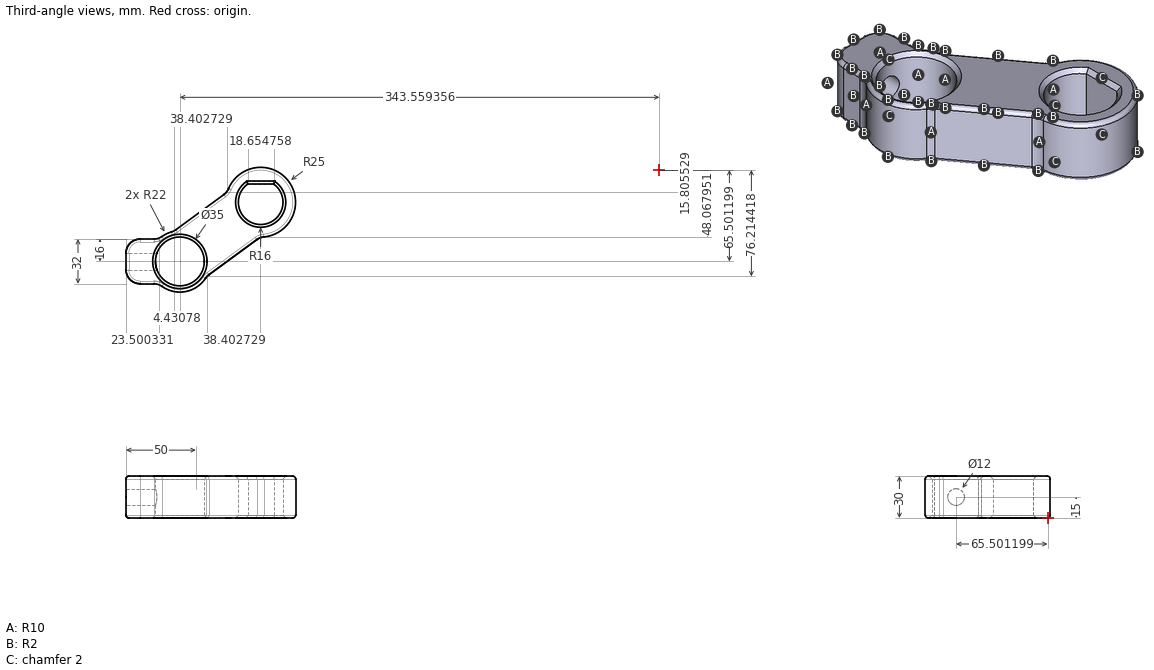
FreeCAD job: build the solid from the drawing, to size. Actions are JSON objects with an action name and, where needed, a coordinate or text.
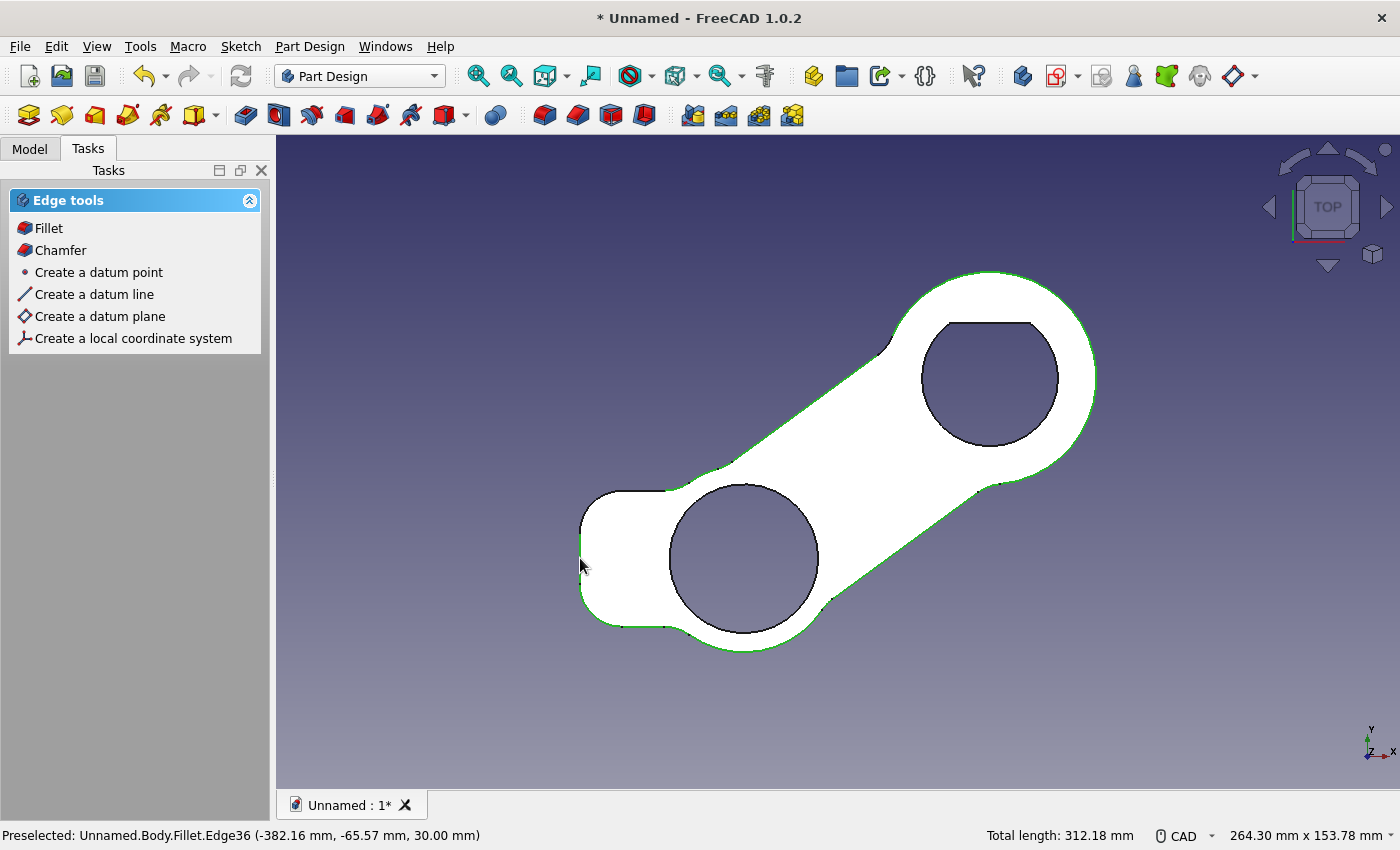
{"action": "left_click", "coordinate": [643, 490], "text": "ctrl"}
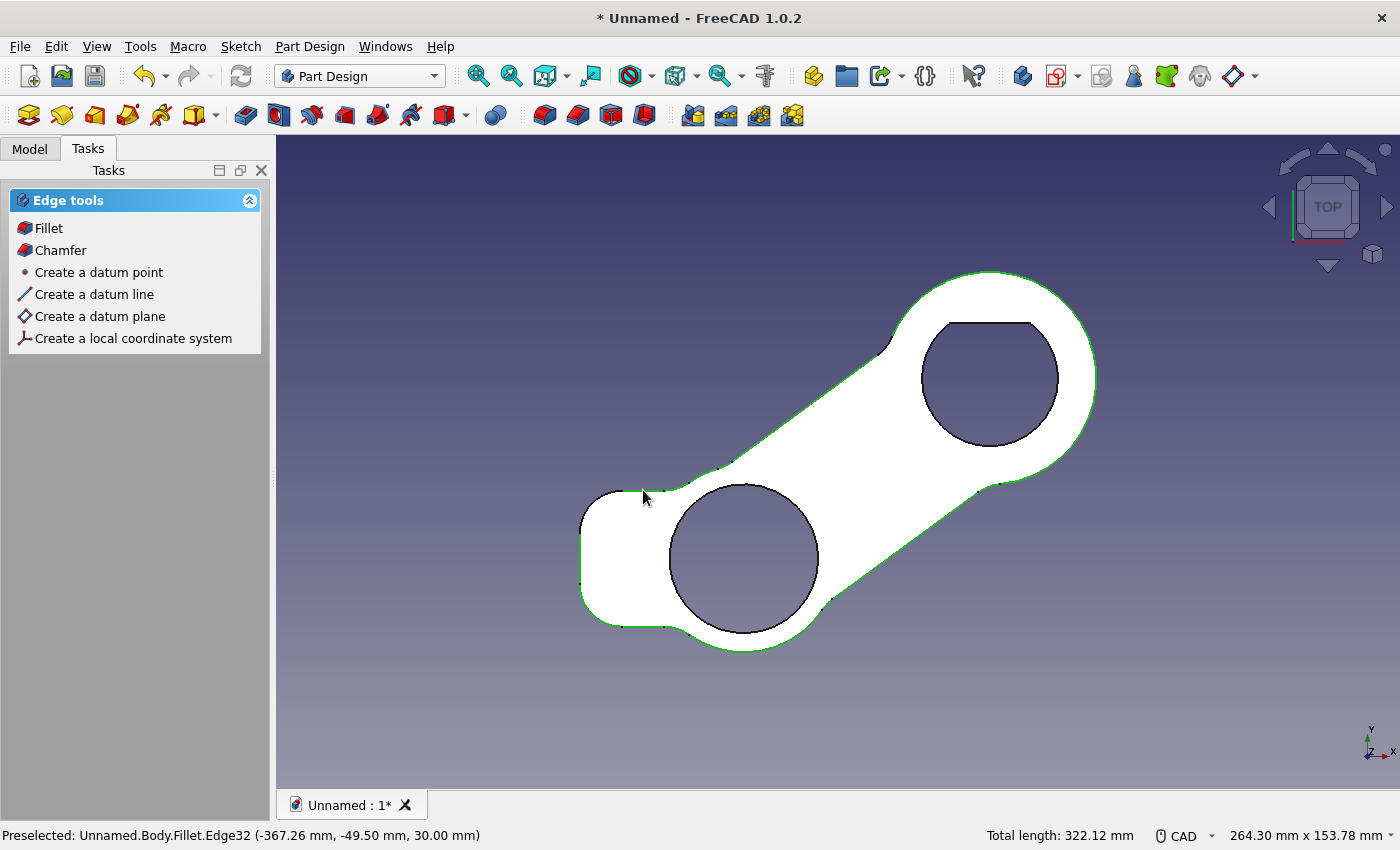
{"action": "left_click", "coordinate": [592, 502], "text": "ctrl"}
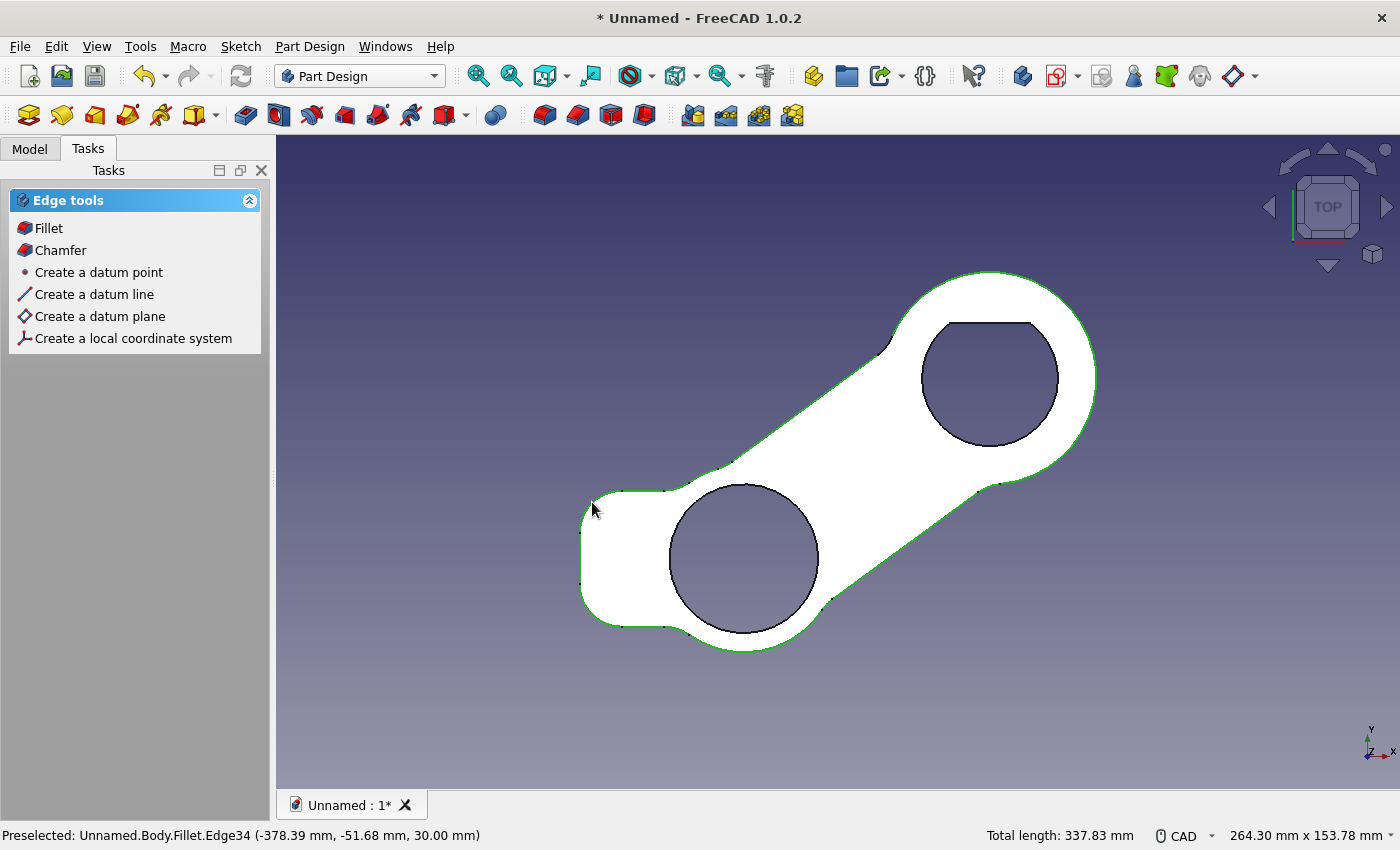
{"action": "left_click", "coordinate": [886, 346], "text": "ctrl"}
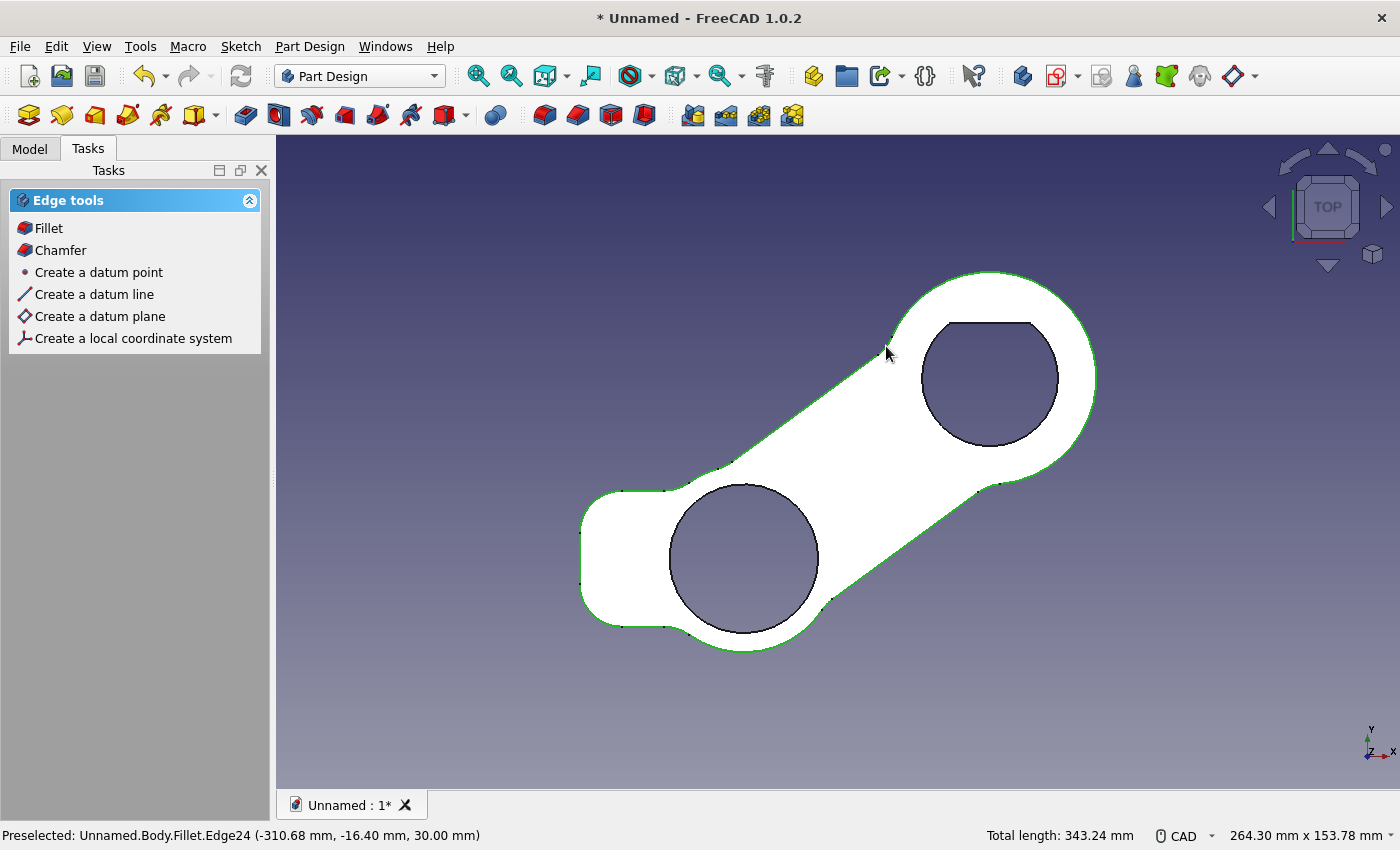
{"action": "key", "text": "0"}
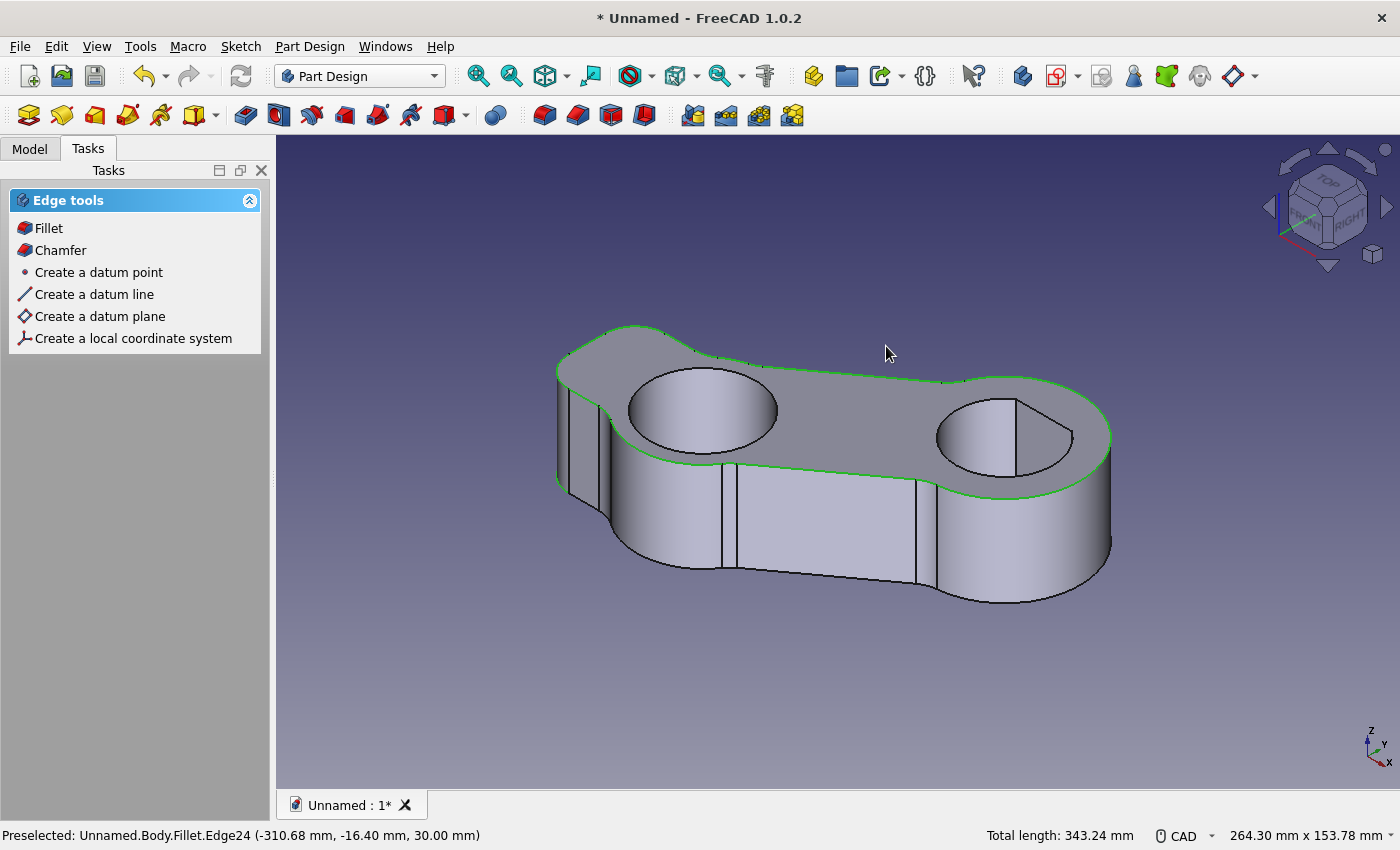
{"action": "key", "text": "1"}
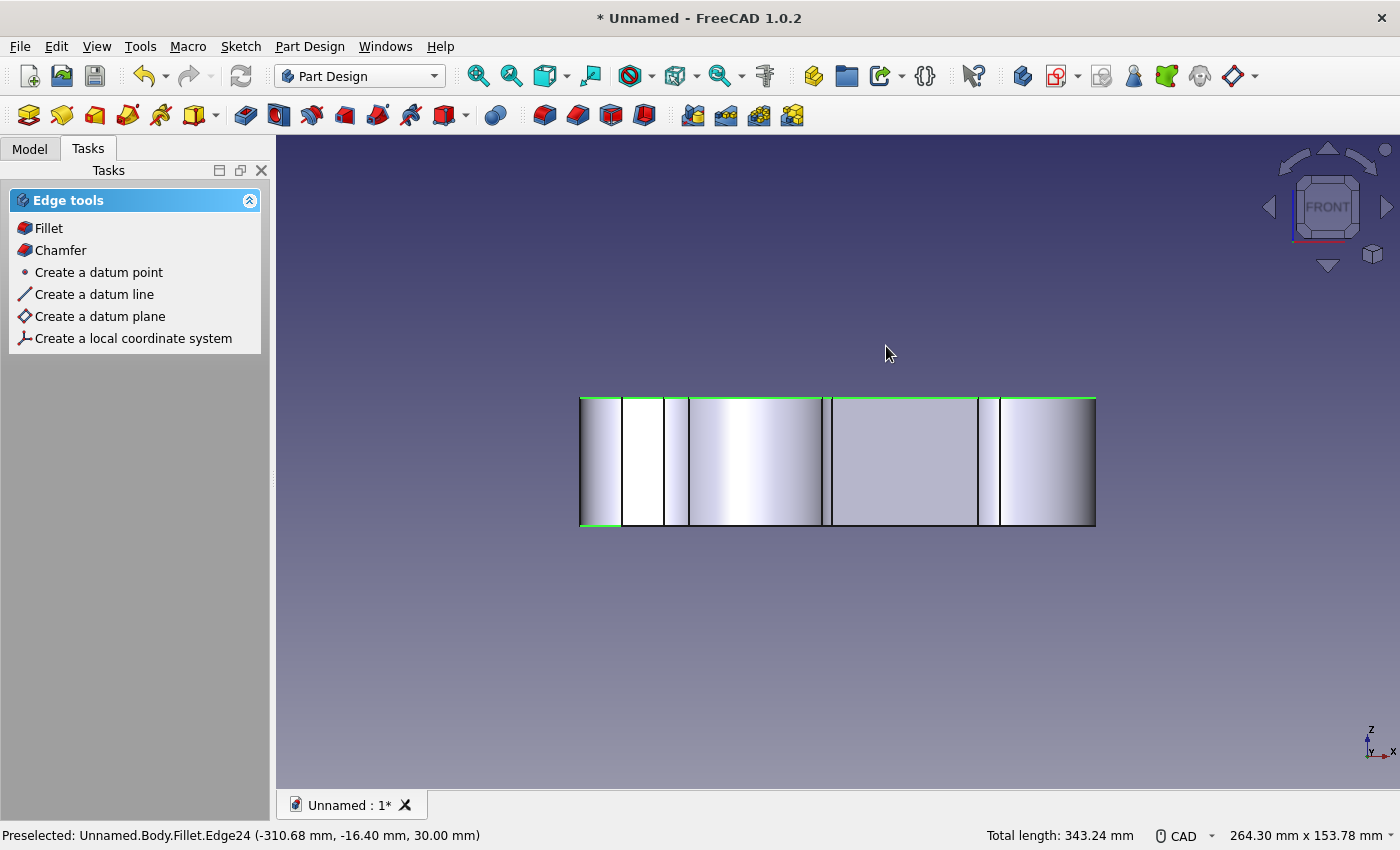
{"action": "left_click", "coordinate": [1076, 525], "text": "ctrl"}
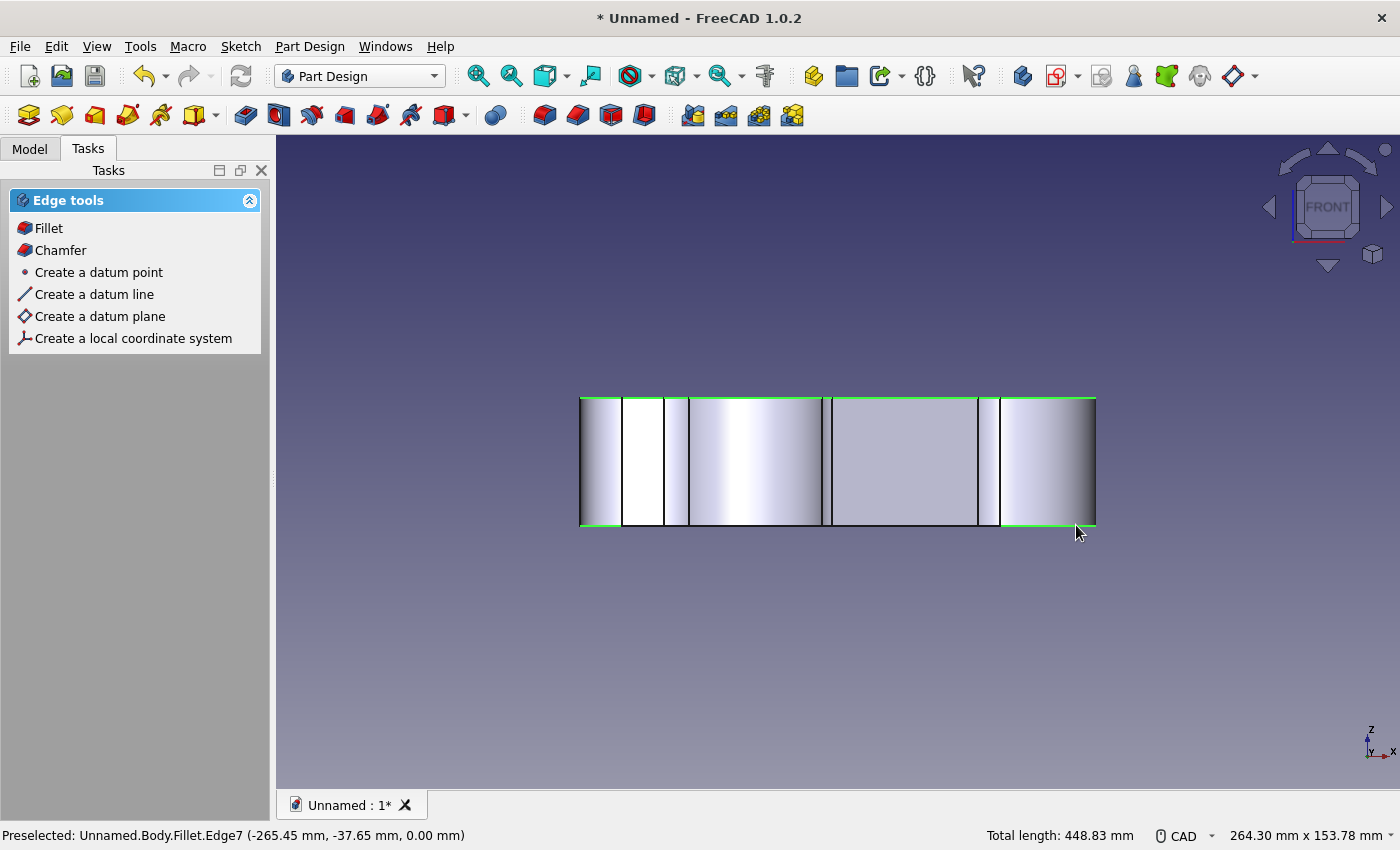
{"action": "left_click", "coordinate": [905, 525], "text": "ctrl"}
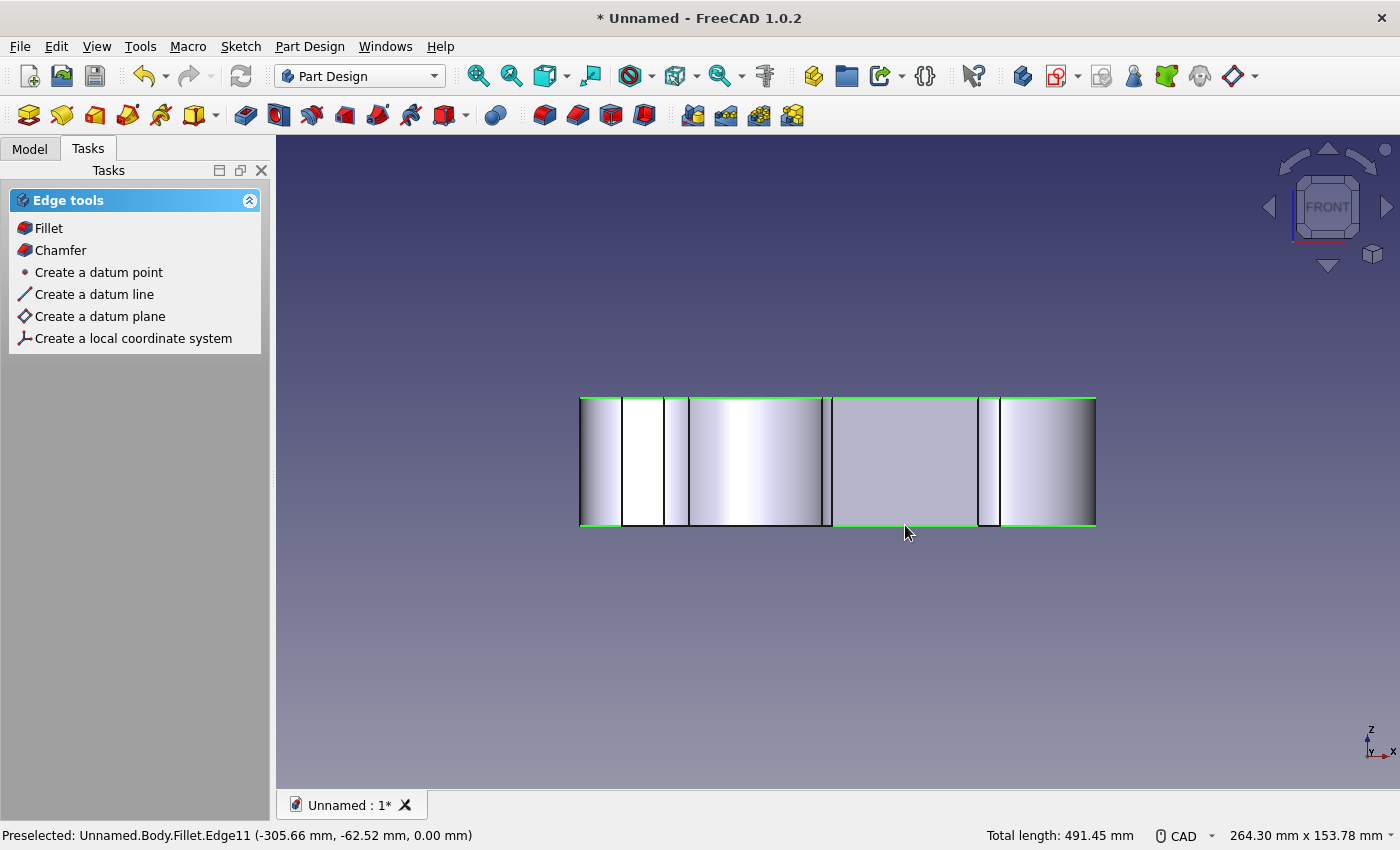
{"action": "left_click", "coordinate": [761, 525], "text": "ctrl"}